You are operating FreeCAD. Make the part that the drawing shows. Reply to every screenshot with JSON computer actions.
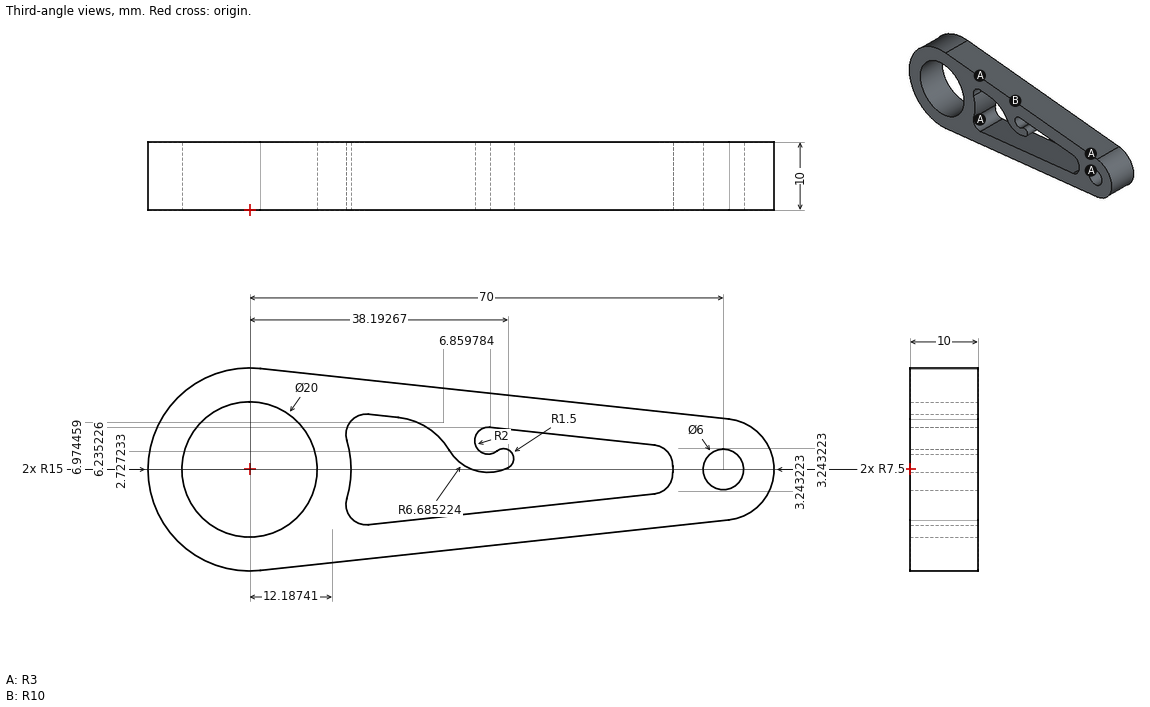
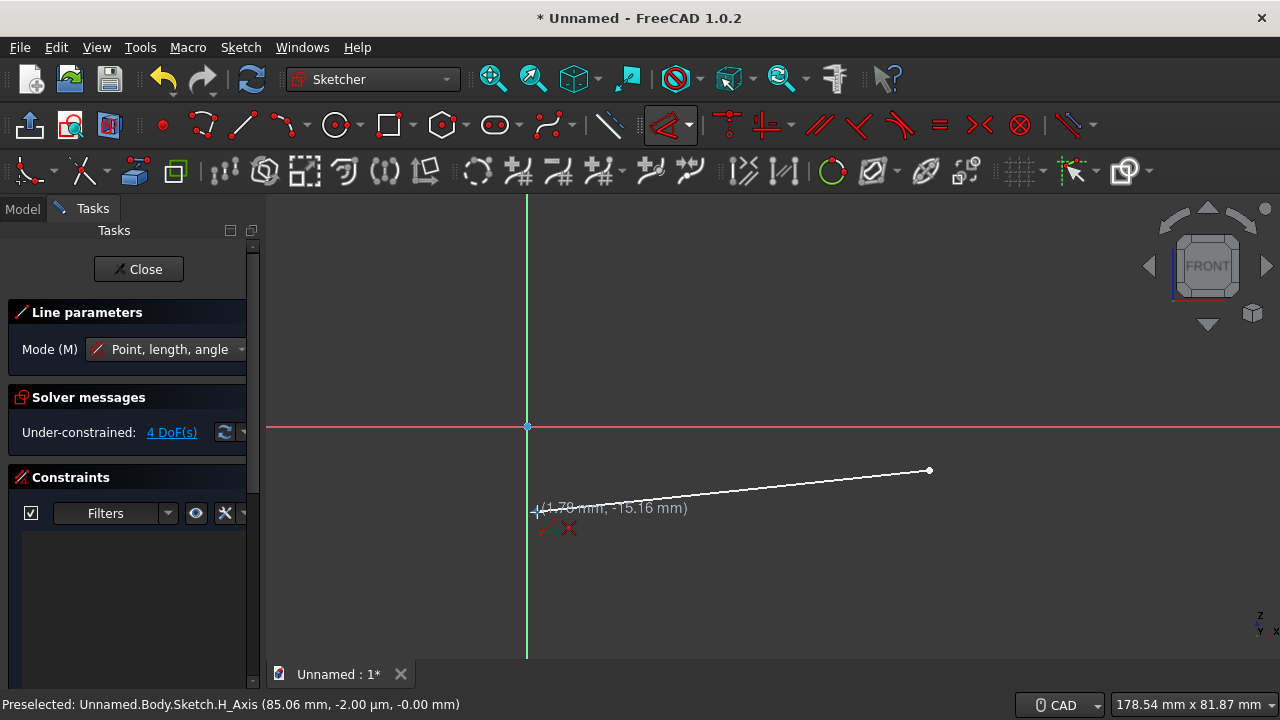
{"action": "scroll", "coordinate": [536, 342], "scroll_direction": "up", "scroll_amount": 3}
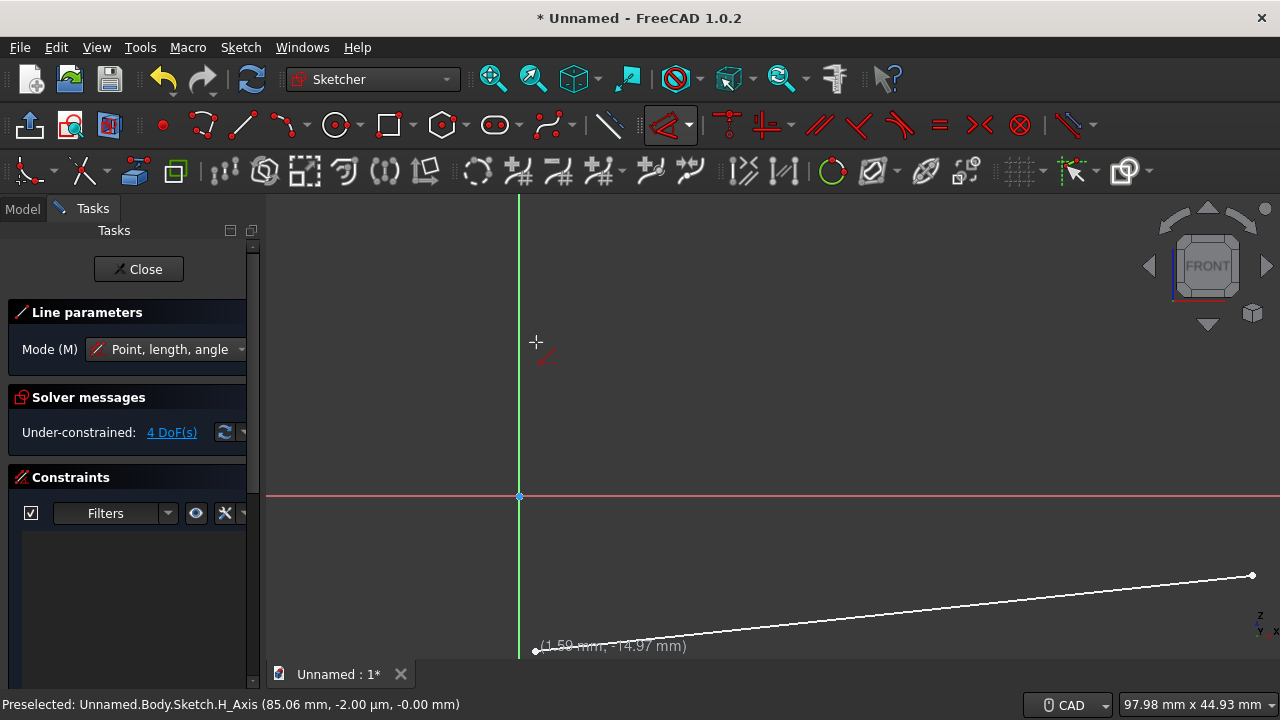
{"action": "left_click", "coordinate": [536, 342]}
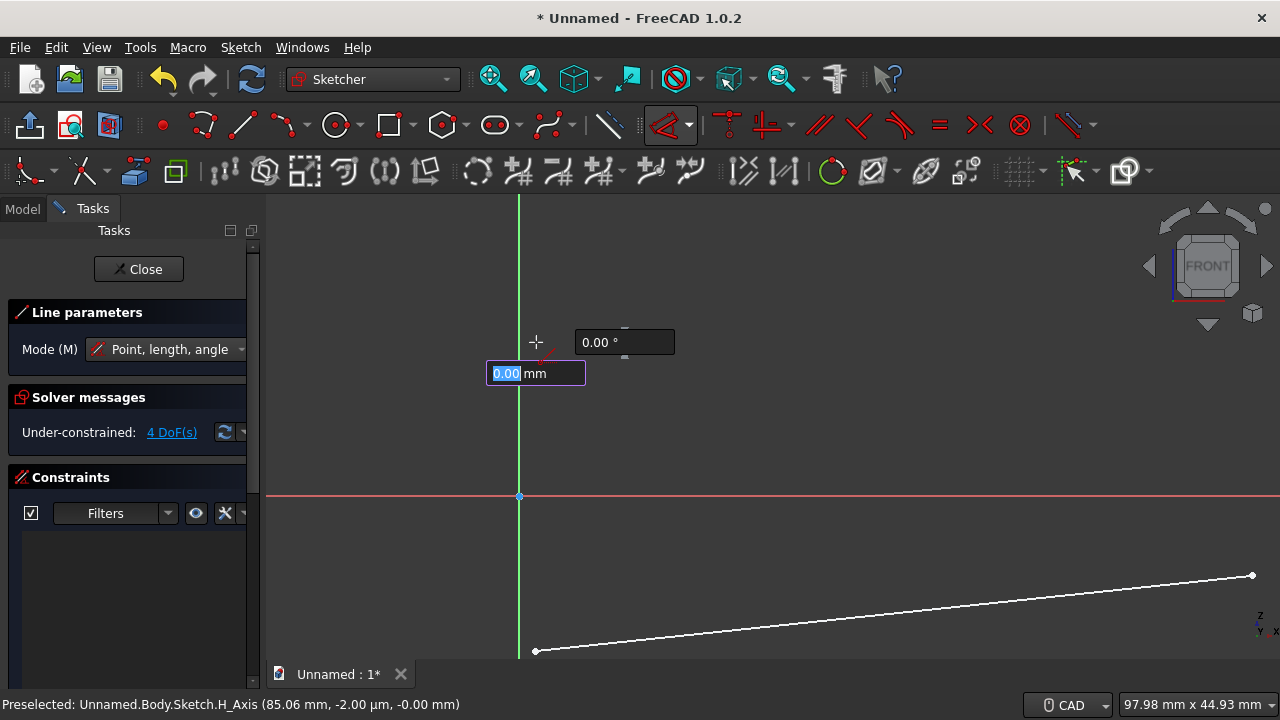
{"action": "scroll", "coordinate": [536, 342], "scroll_direction": "down", "scroll_amount": 3}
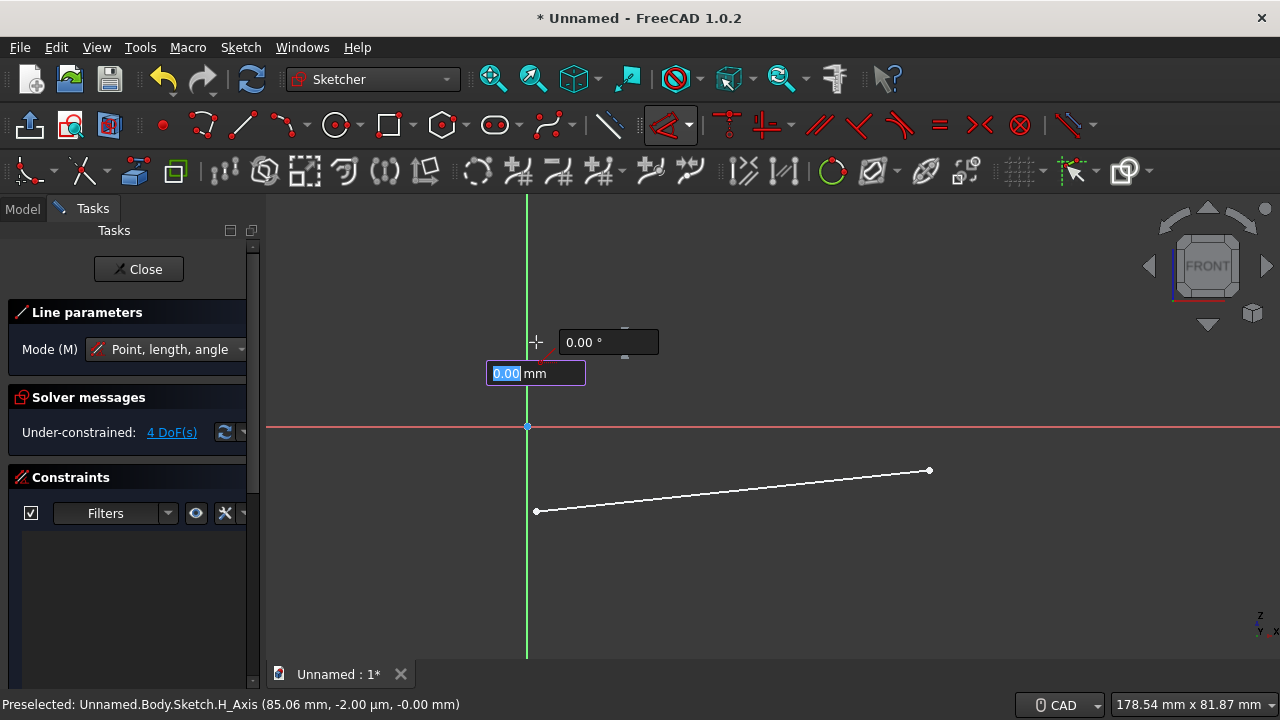
{"action": "left_click", "coordinate": [929, 384]}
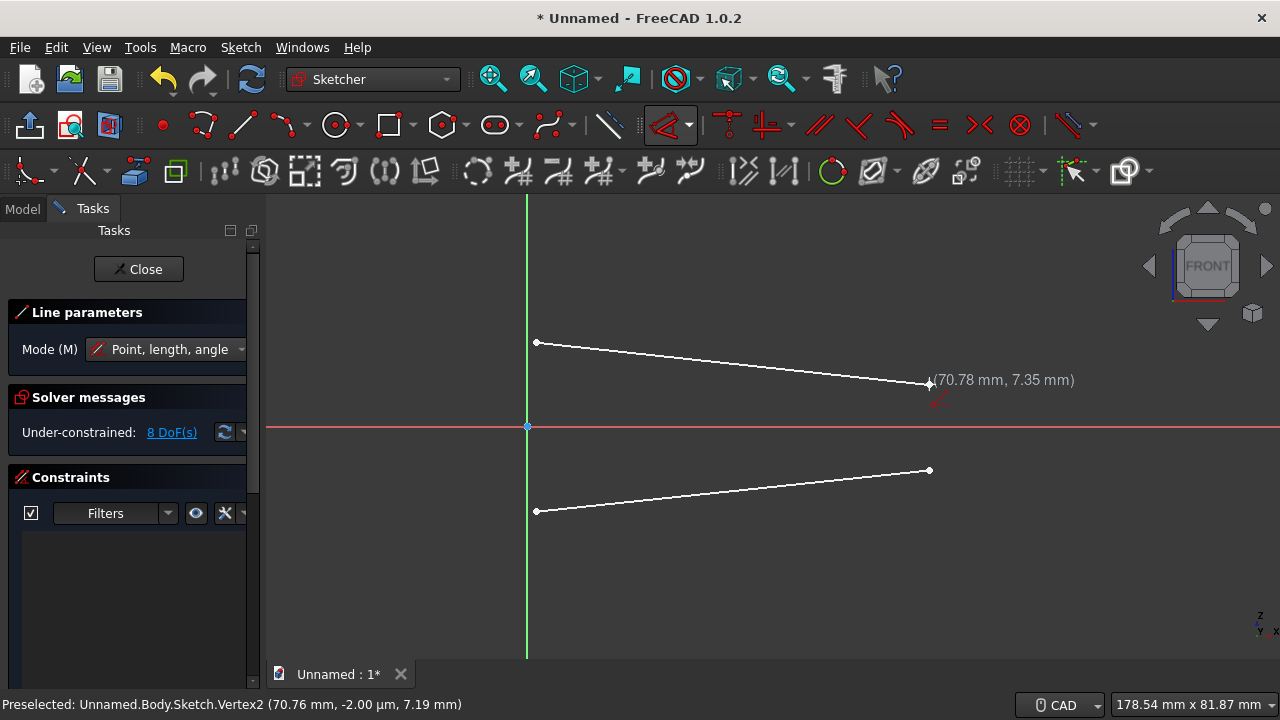
{"action": "key", "text": "g 3 a"}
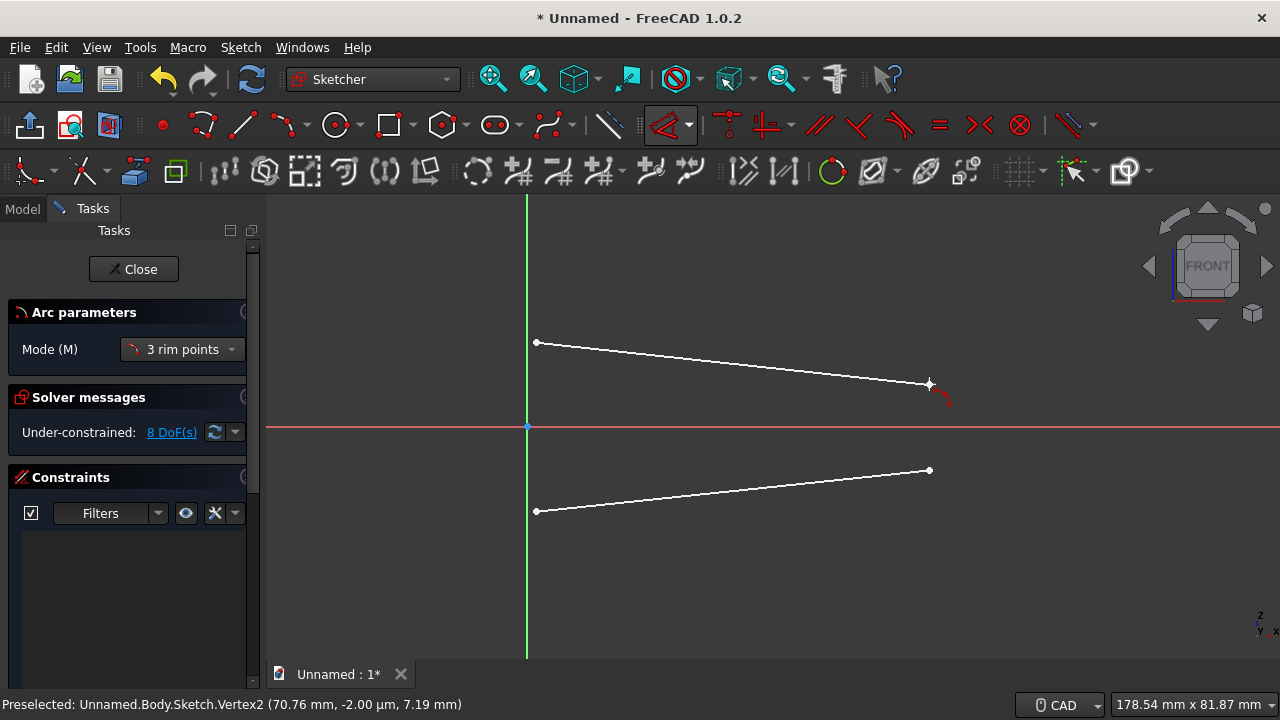
{"action": "scroll", "coordinate": [536, 511], "scroll_direction": "up", "scroll_amount": 3}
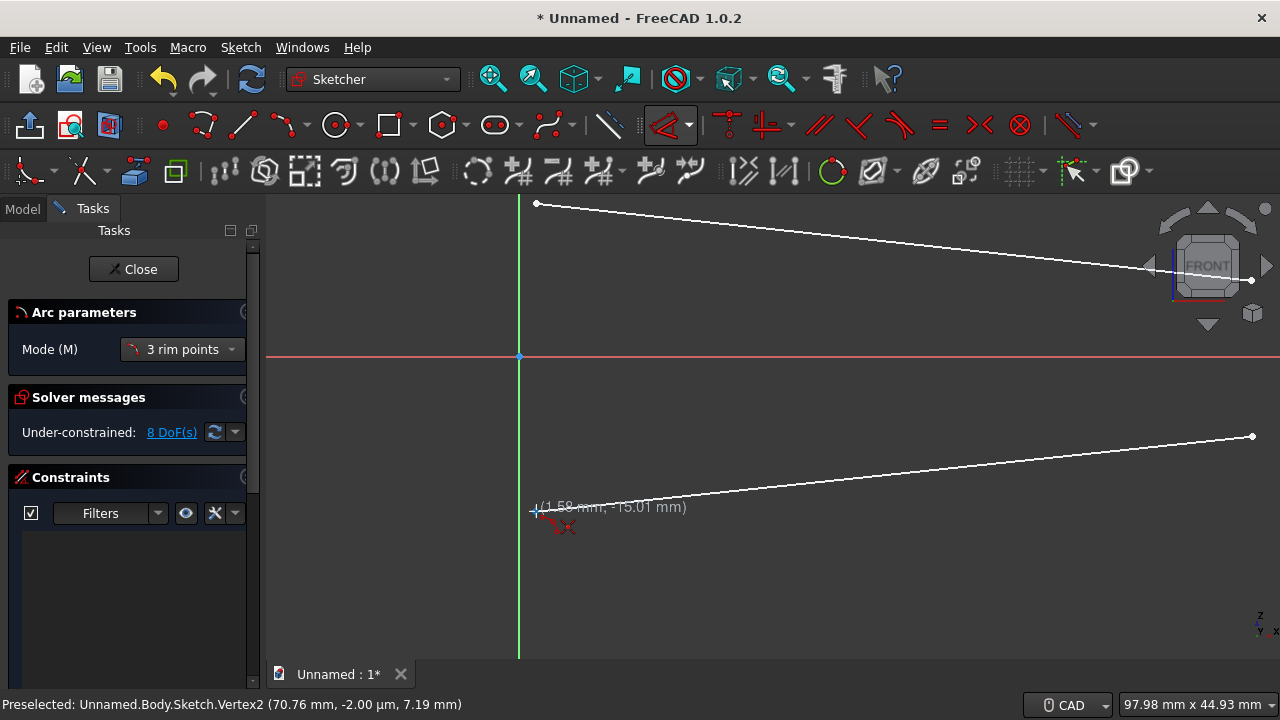
{"action": "left_click", "coordinate": [536, 512]}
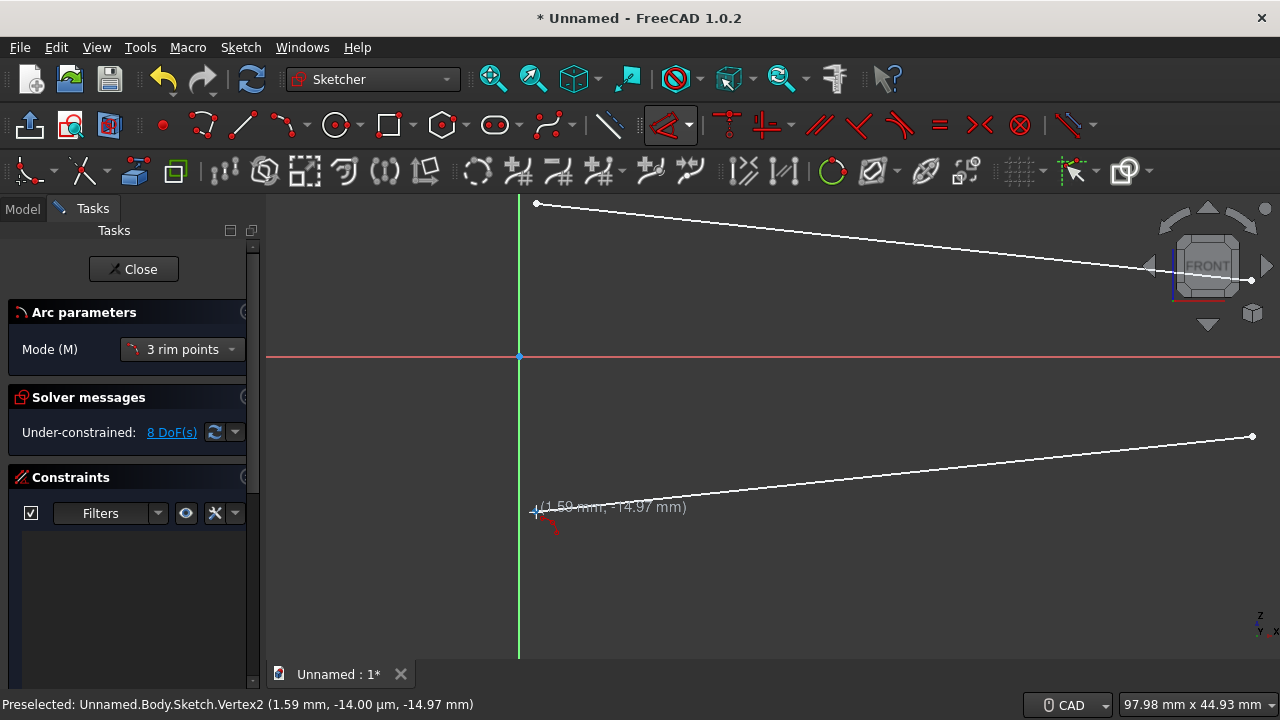
{"action": "scroll", "coordinate": [536, 511], "scroll_direction": "down", "scroll_amount": 3}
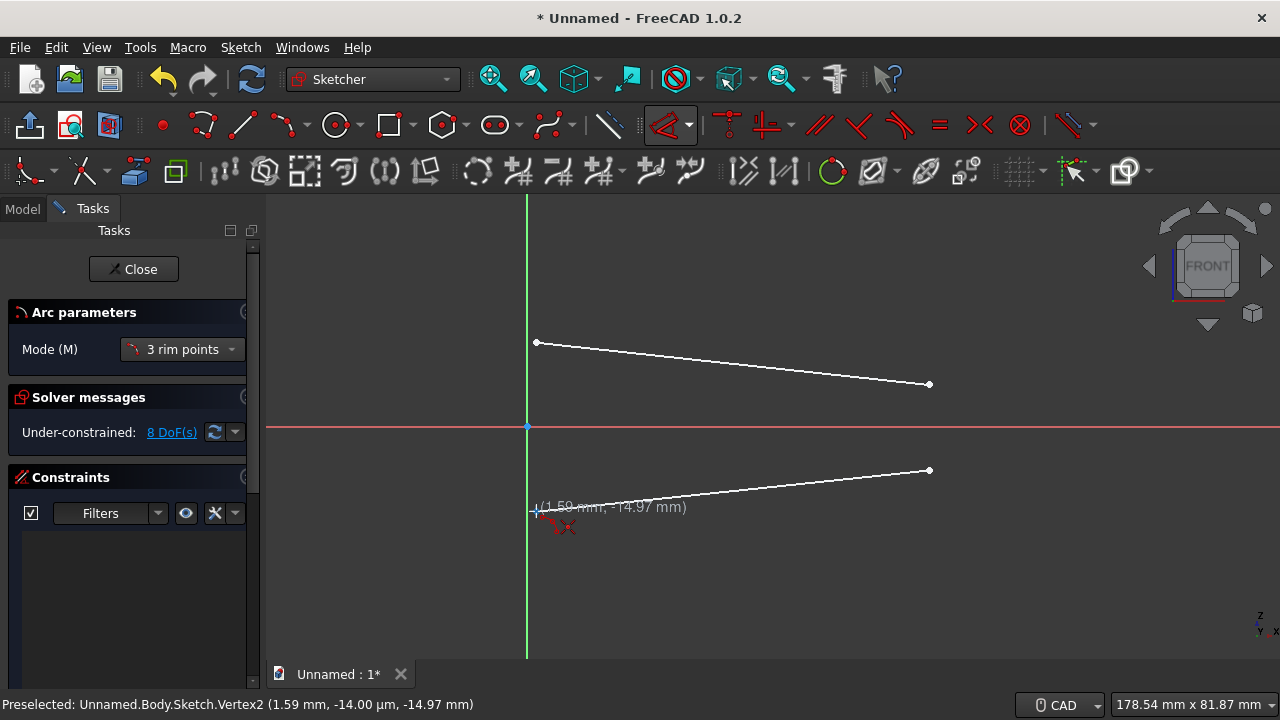
{"action": "scroll", "coordinate": [536, 342], "scroll_direction": "up", "scroll_amount": 3}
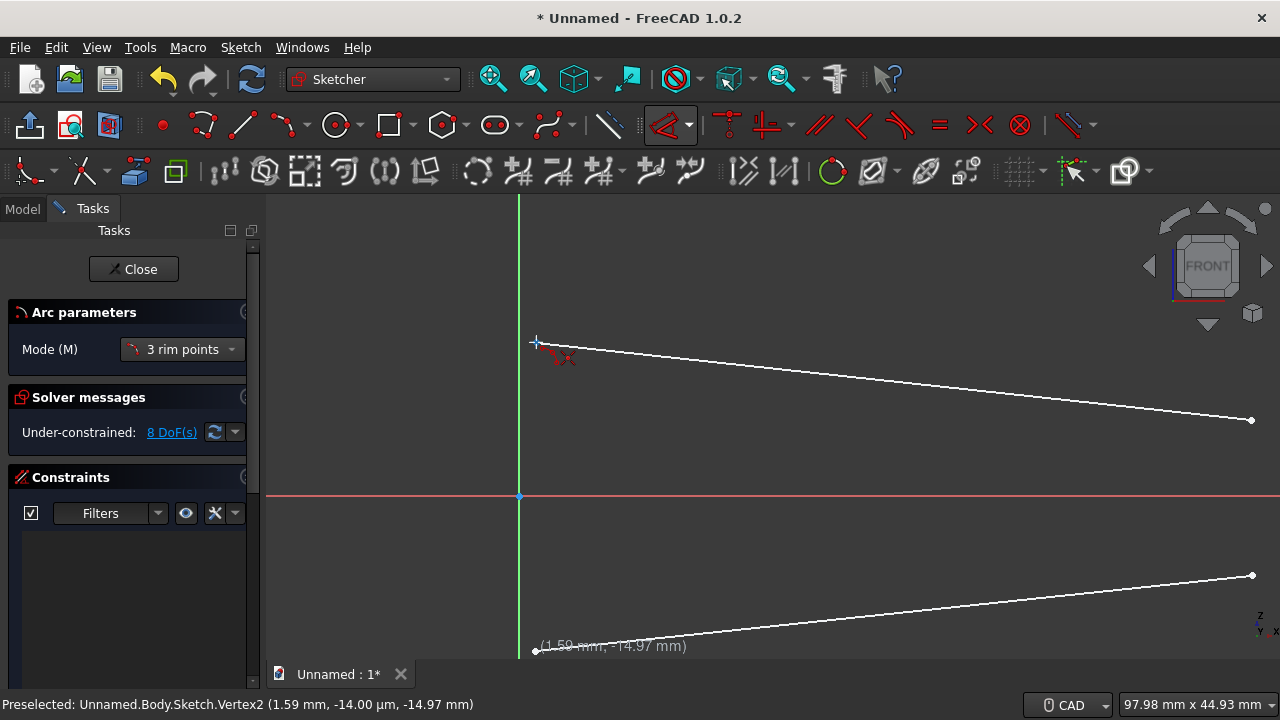
{"action": "left_click", "coordinate": [536, 343]}
{"action": "left_click", "coordinate": [373, 445]}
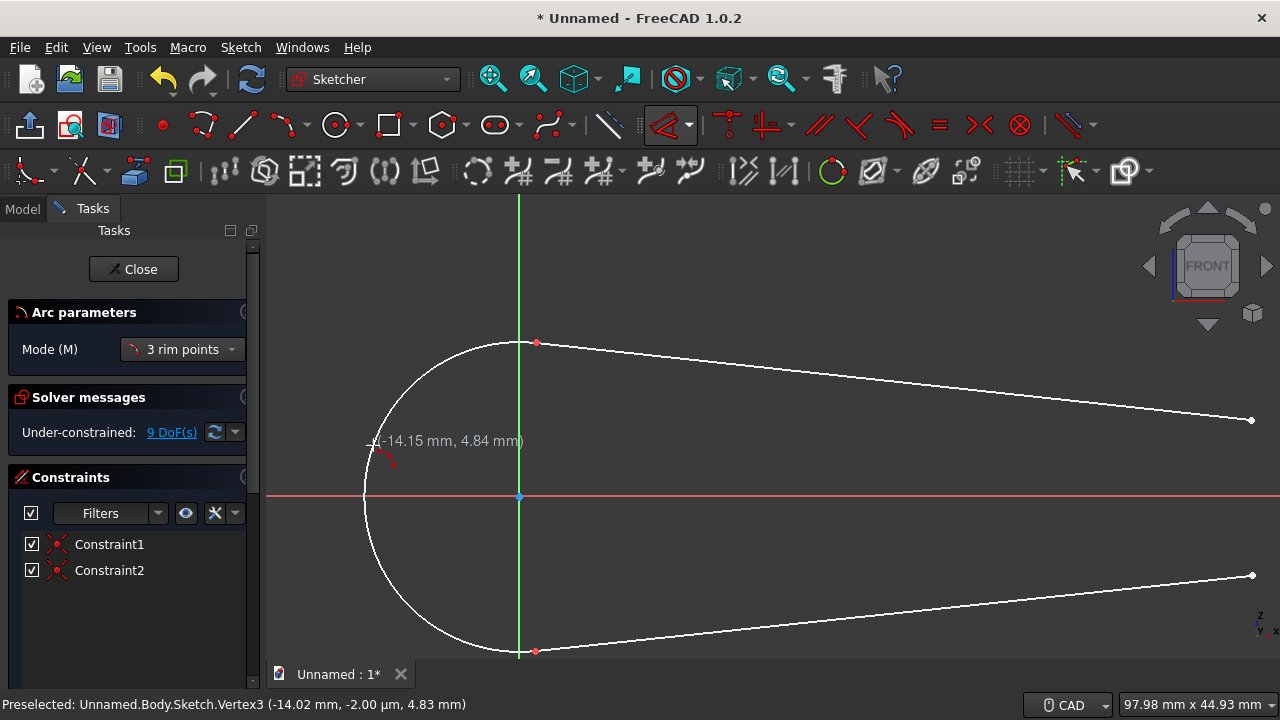
{"action": "scroll", "coordinate": [536, 342], "scroll_direction": "down", "scroll_amount": 3}